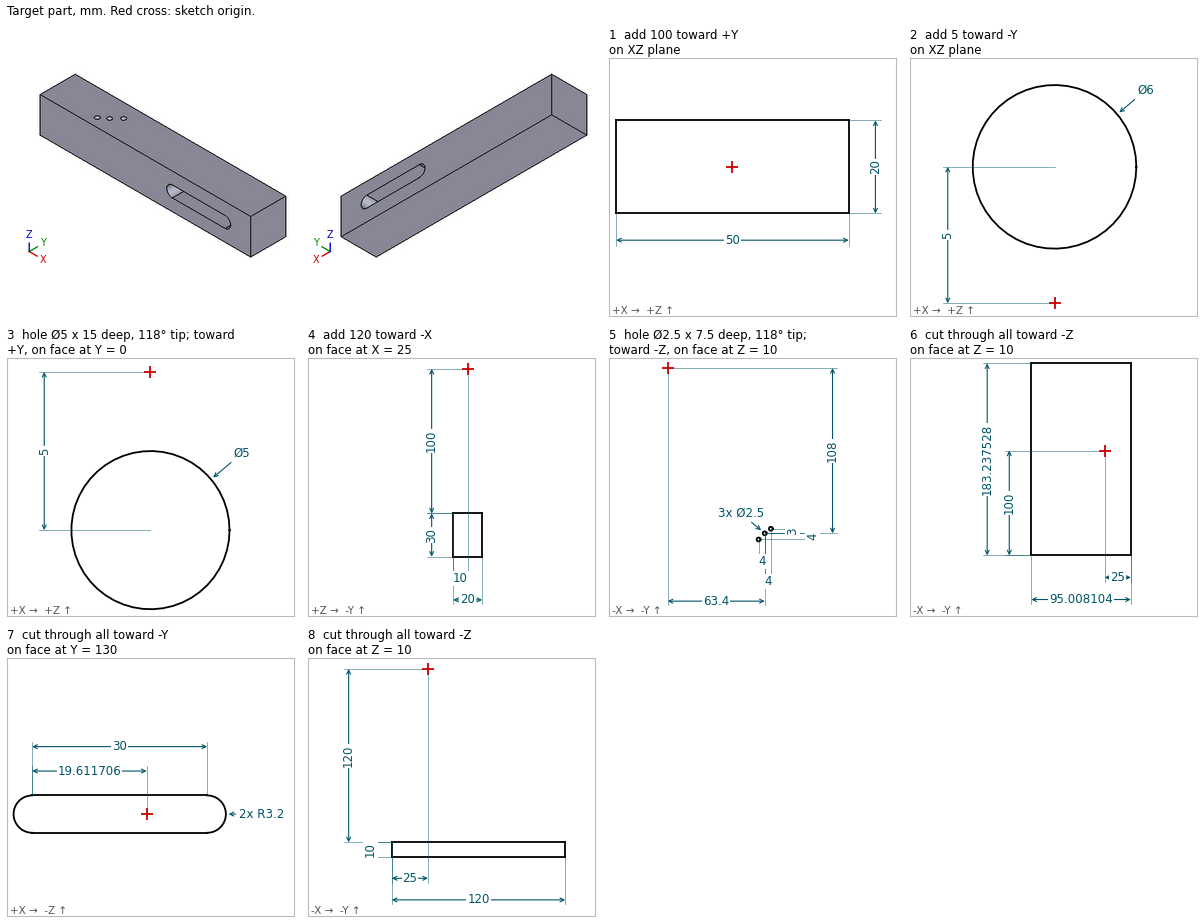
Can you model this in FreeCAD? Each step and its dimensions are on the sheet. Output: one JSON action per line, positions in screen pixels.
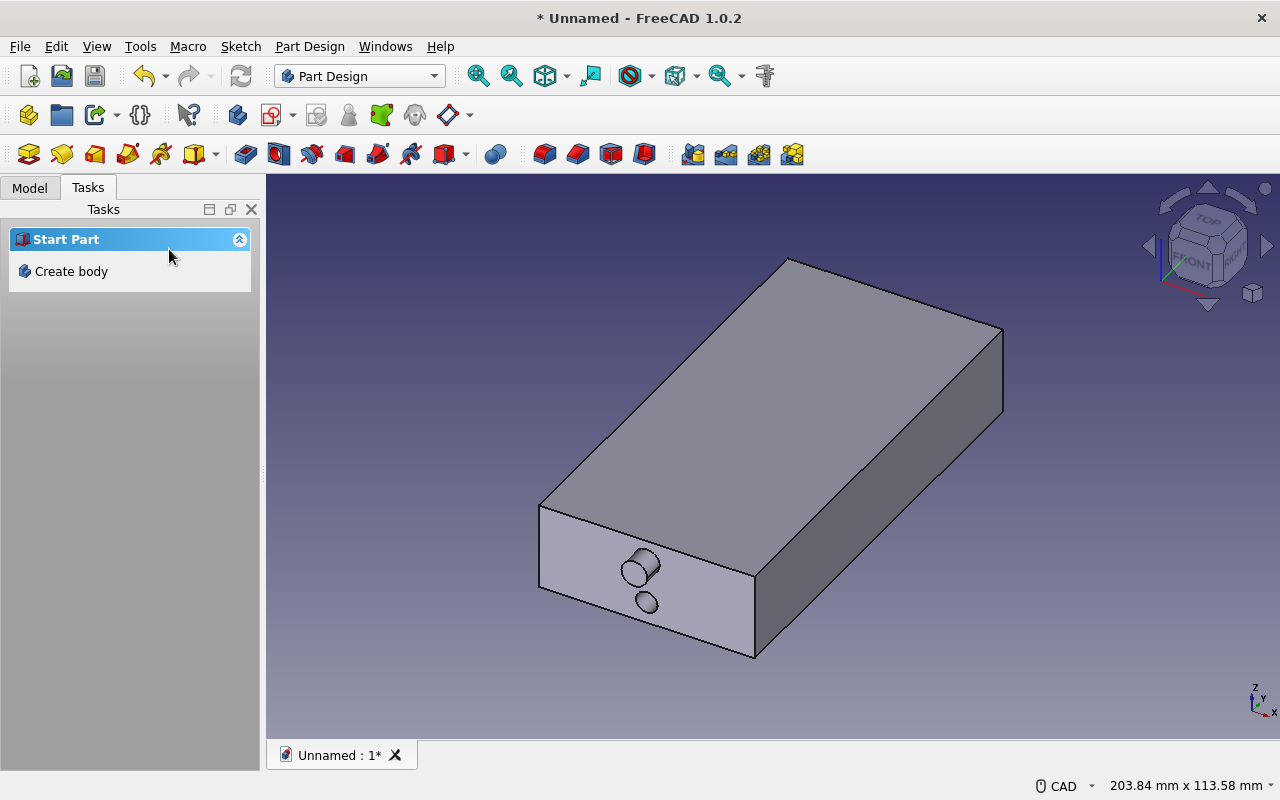
{"action": "left_click", "coordinate": [950, 422]}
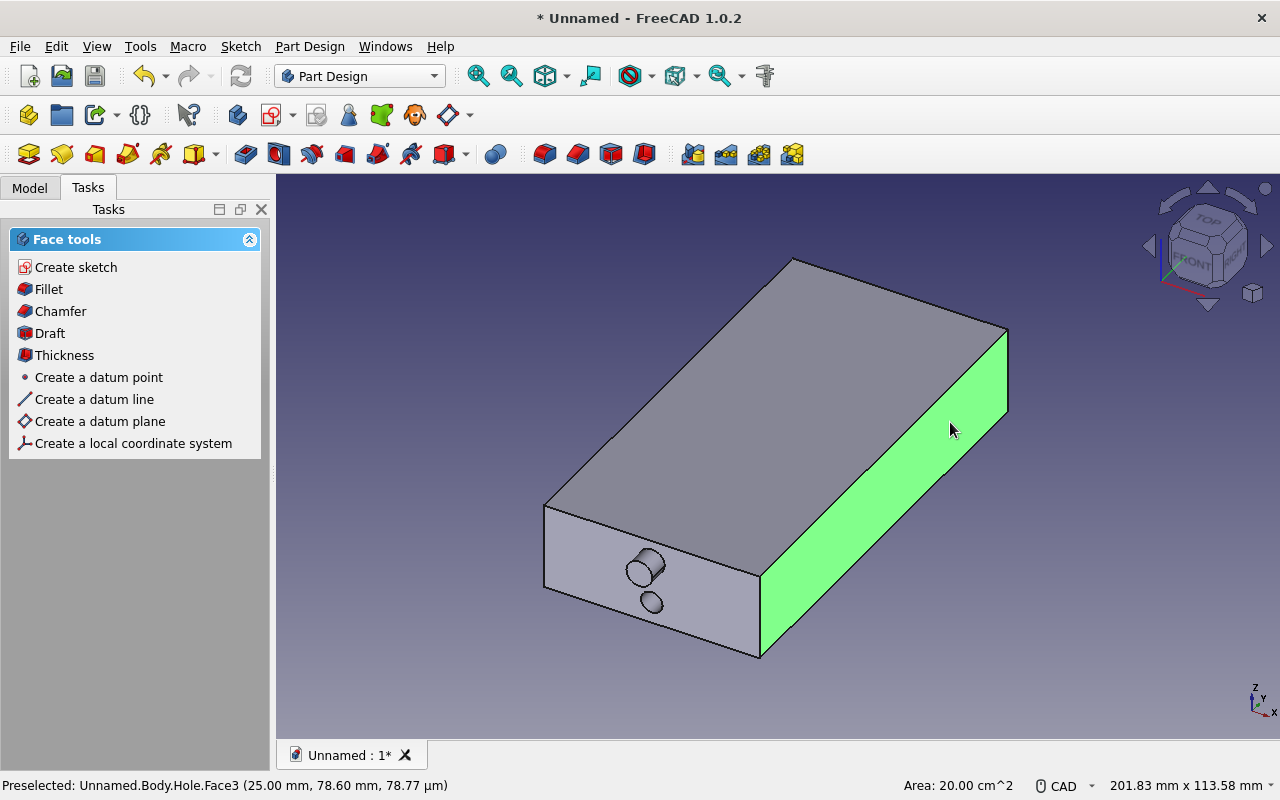
{"action": "left_click", "coordinate": [270, 116]}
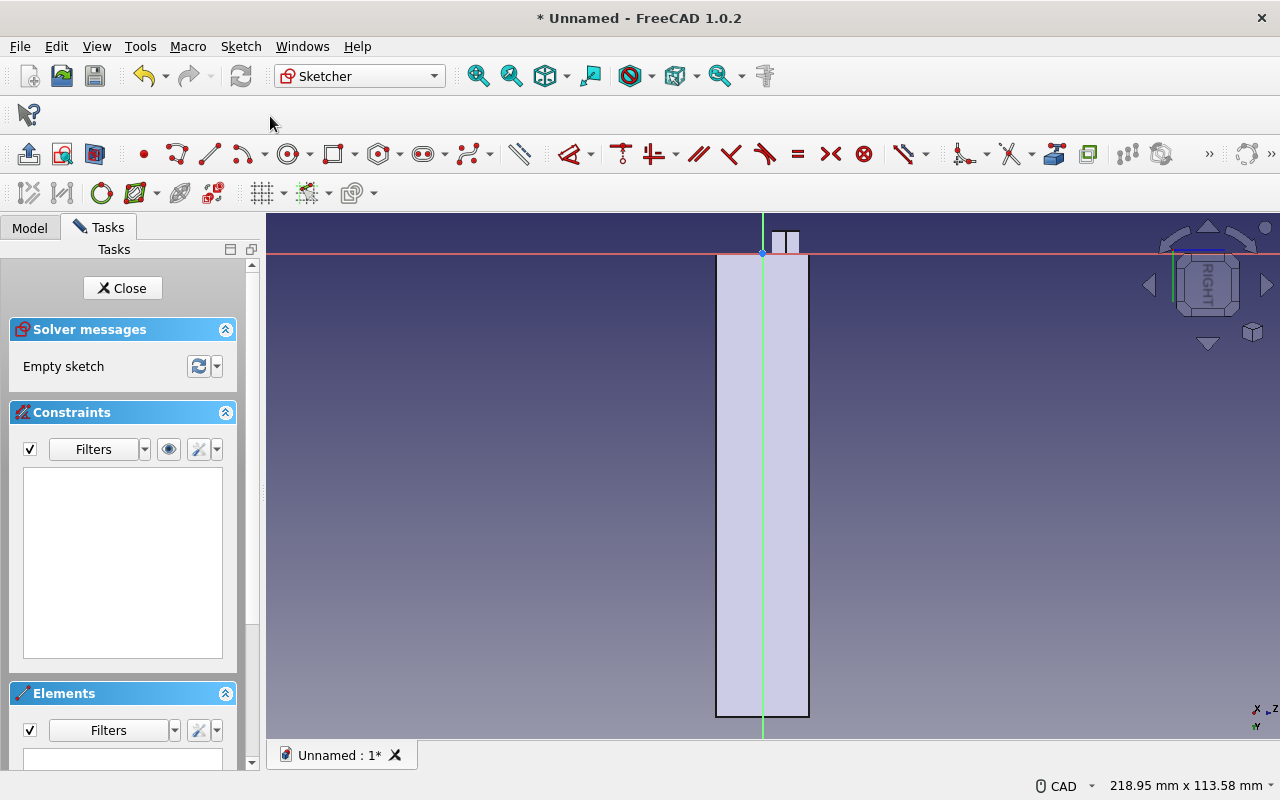
{"action": "scroll", "coordinate": [704, 476], "scroll_direction": "down", "scroll_amount": 5}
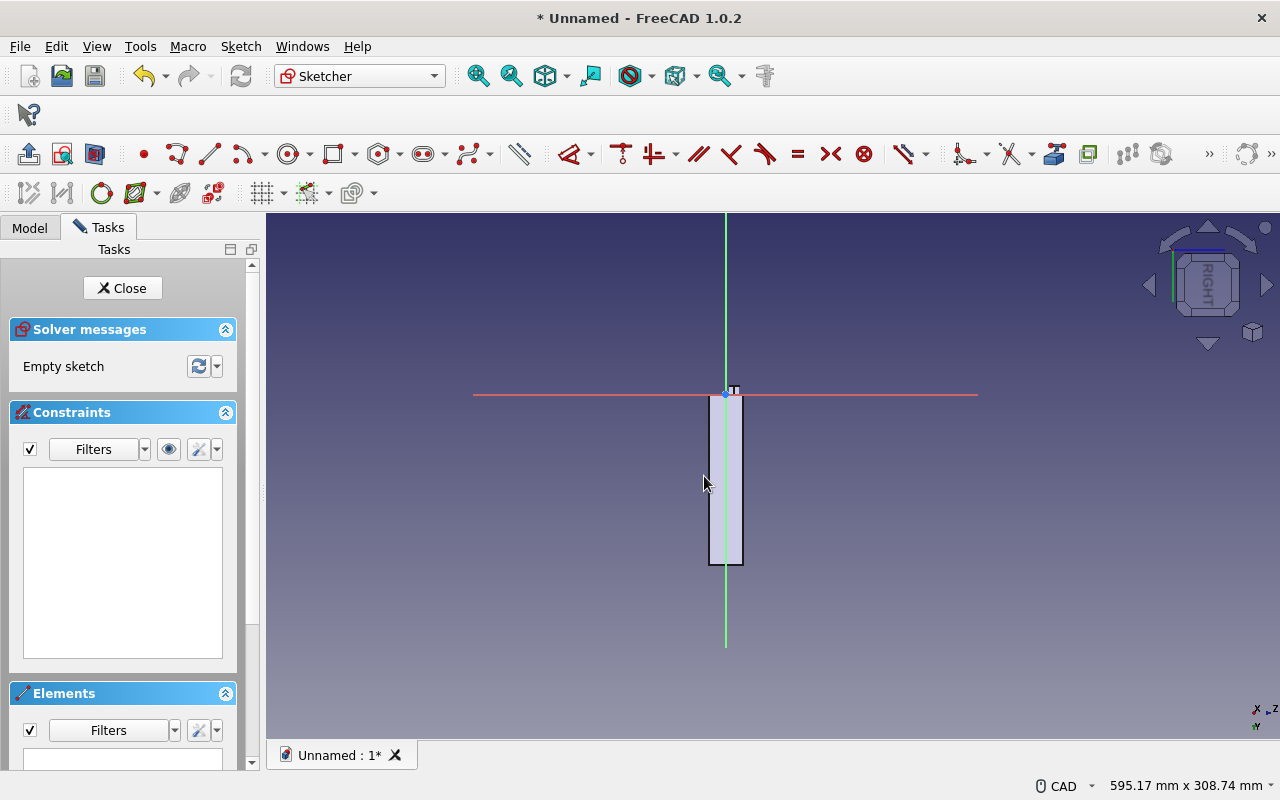
{"action": "scroll", "coordinate": [730, 613], "scroll_direction": "up", "scroll_amount": 9}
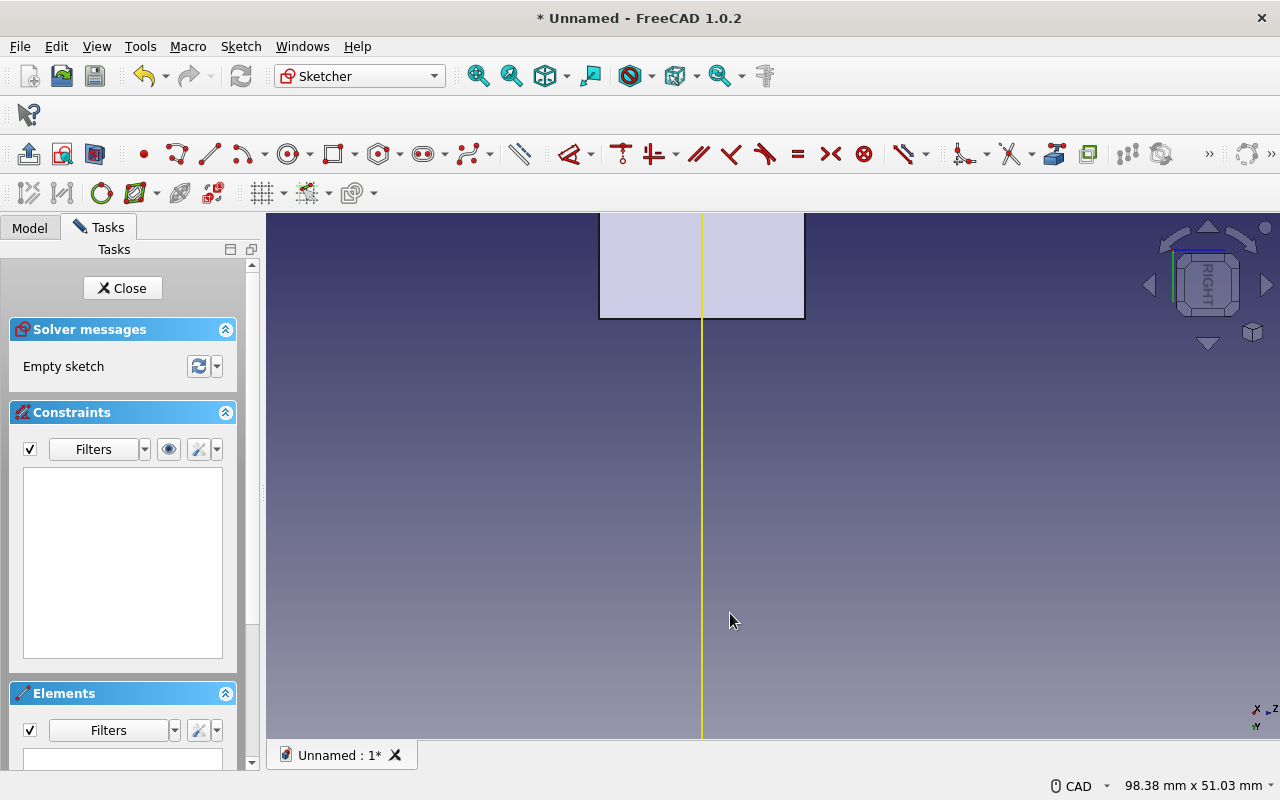
{"action": "left_click", "coordinate": [332, 154]}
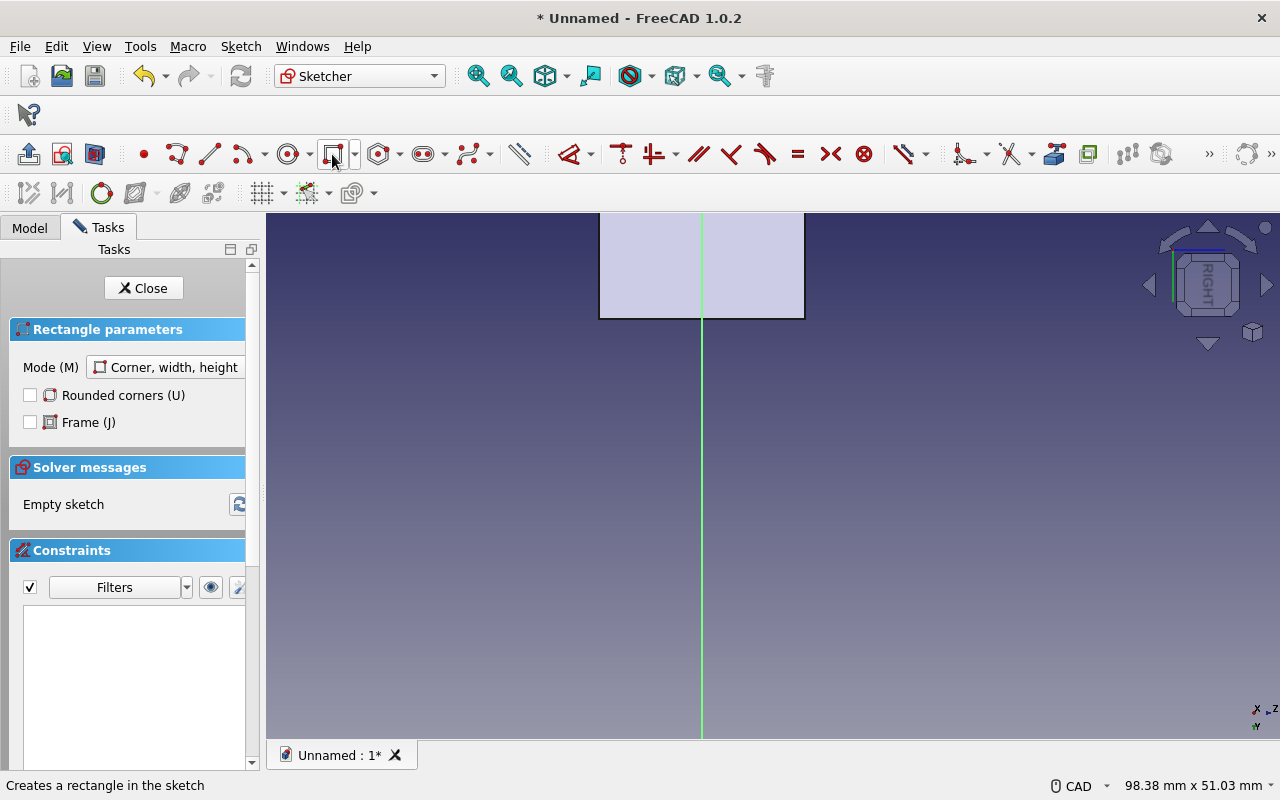
{"action": "left_click", "coordinate": [599, 319]}
{"action": "left_click", "coordinate": [805, 628]}
{"action": "key", "text": "Escape"}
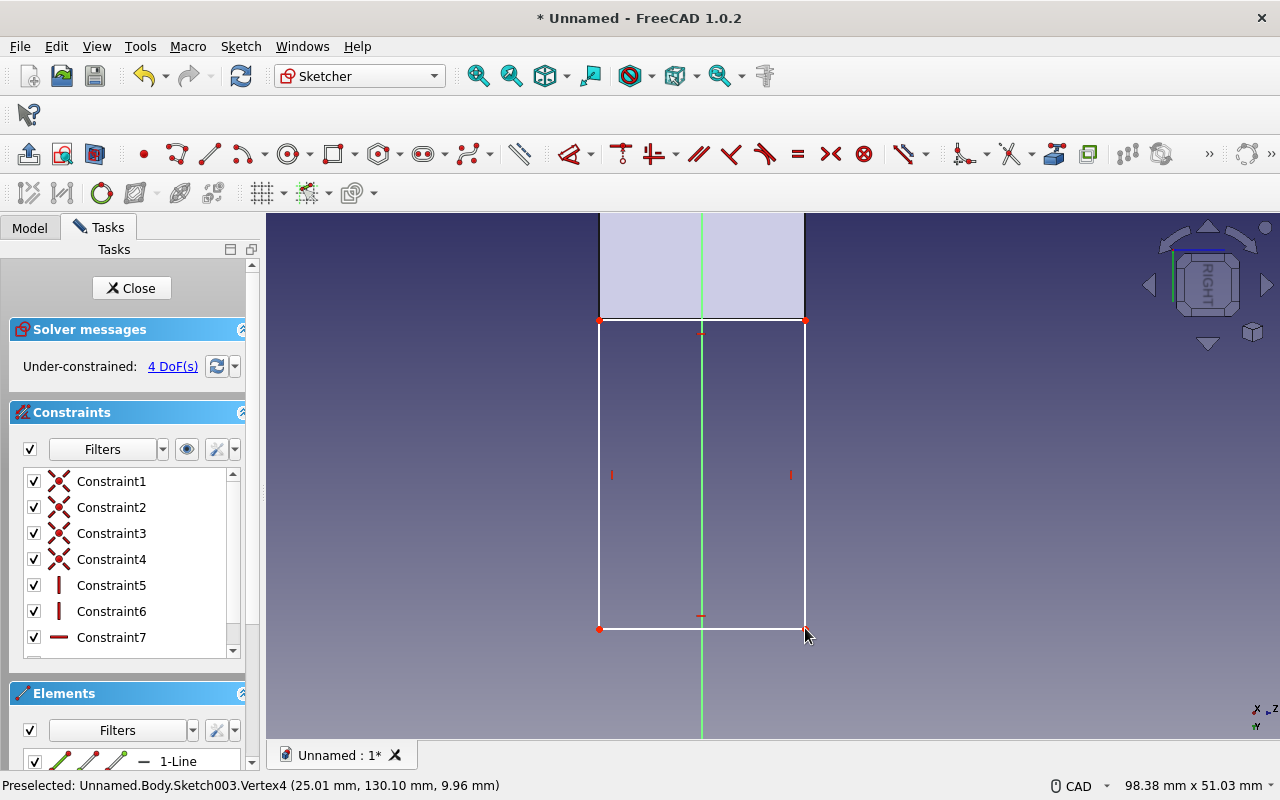
{"action": "left_click", "coordinate": [568, 154]}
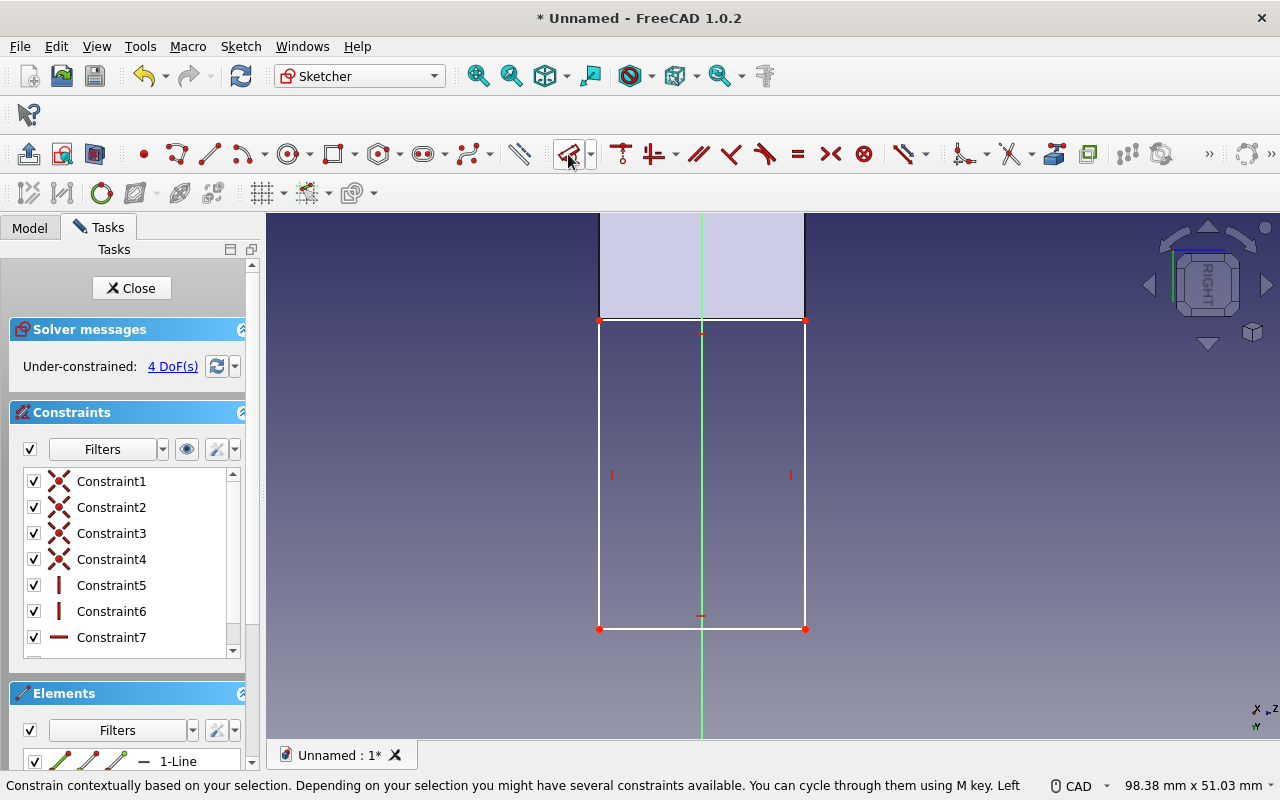
{"action": "left_click", "coordinate": [599, 413]}
{"action": "left_click", "coordinate": [565, 474]}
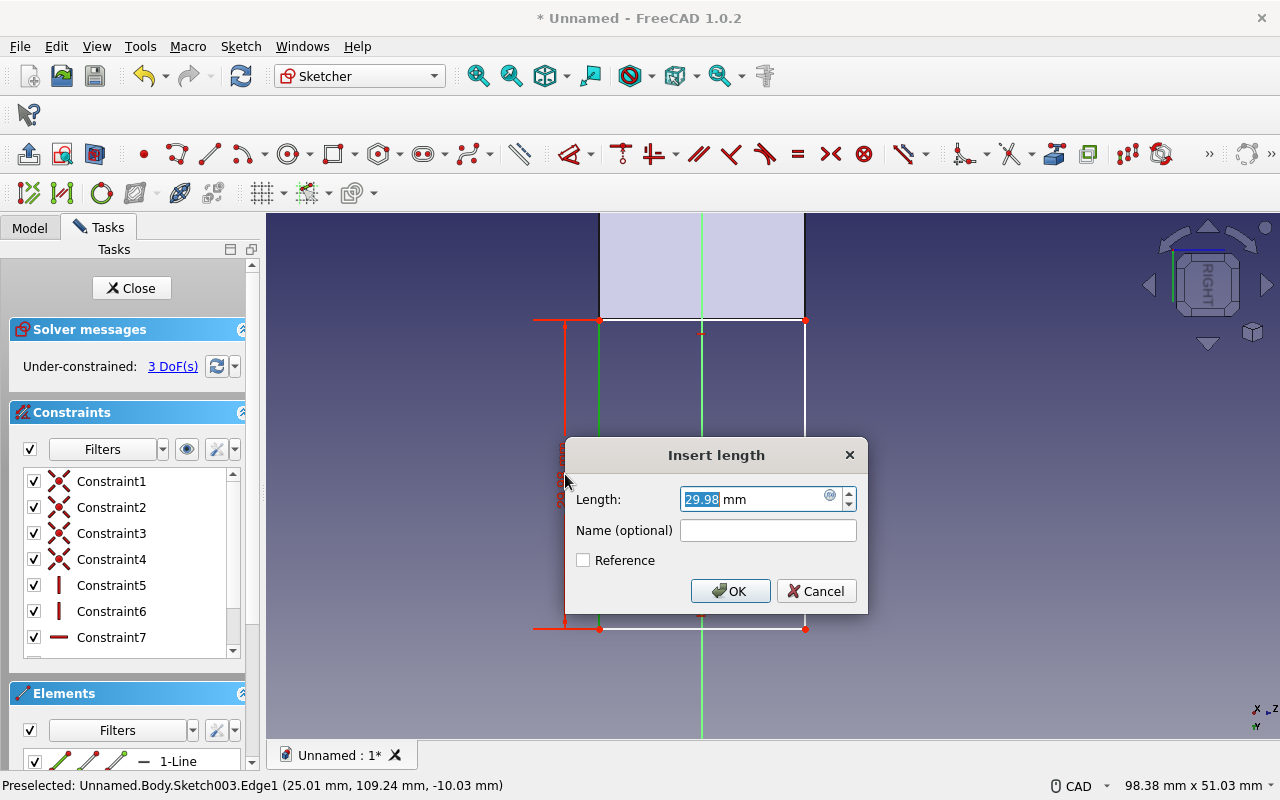
{"action": "type", "text": "30"}
{"action": "key", "text": "Return"}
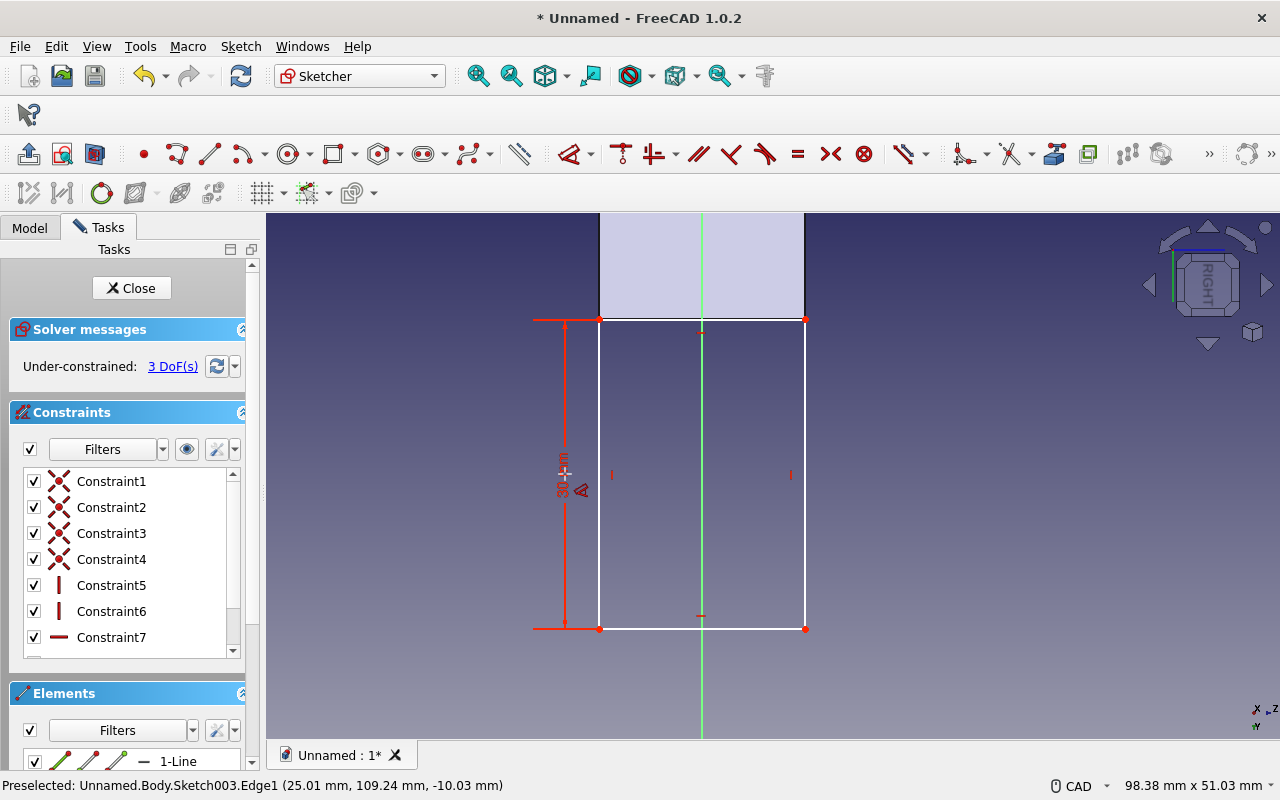
{"action": "left_click", "coordinate": [661, 629]}
{"action": "left_click", "coordinate": [655, 663]}